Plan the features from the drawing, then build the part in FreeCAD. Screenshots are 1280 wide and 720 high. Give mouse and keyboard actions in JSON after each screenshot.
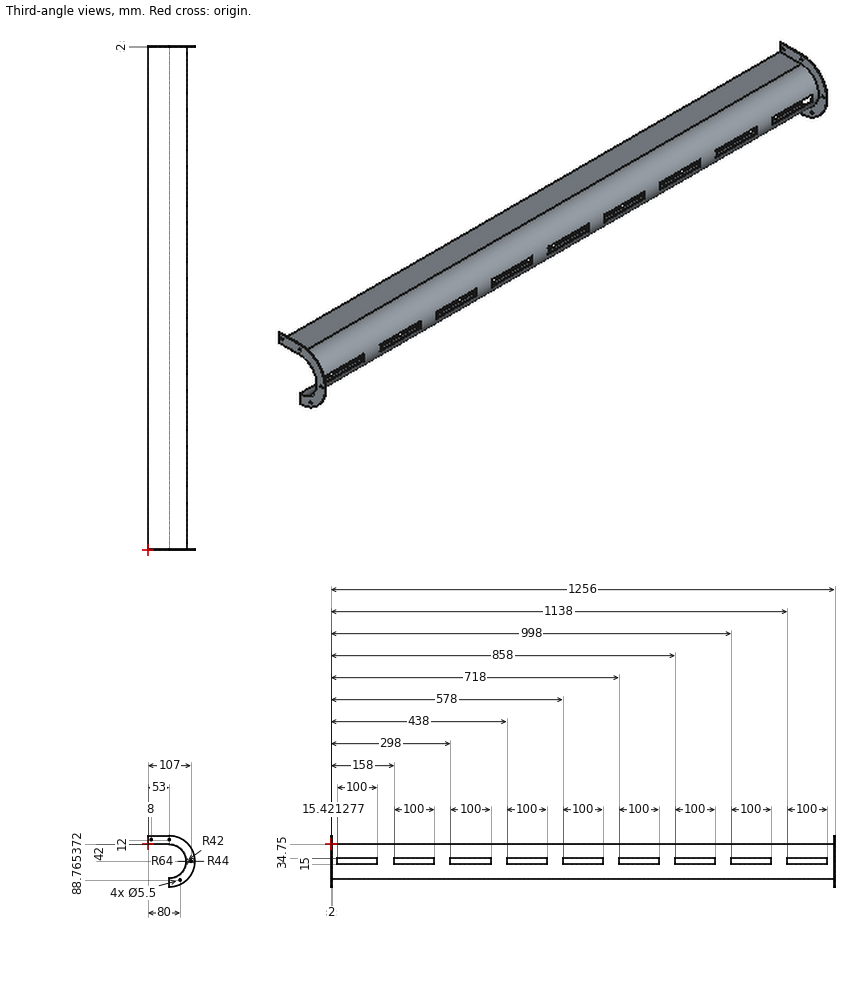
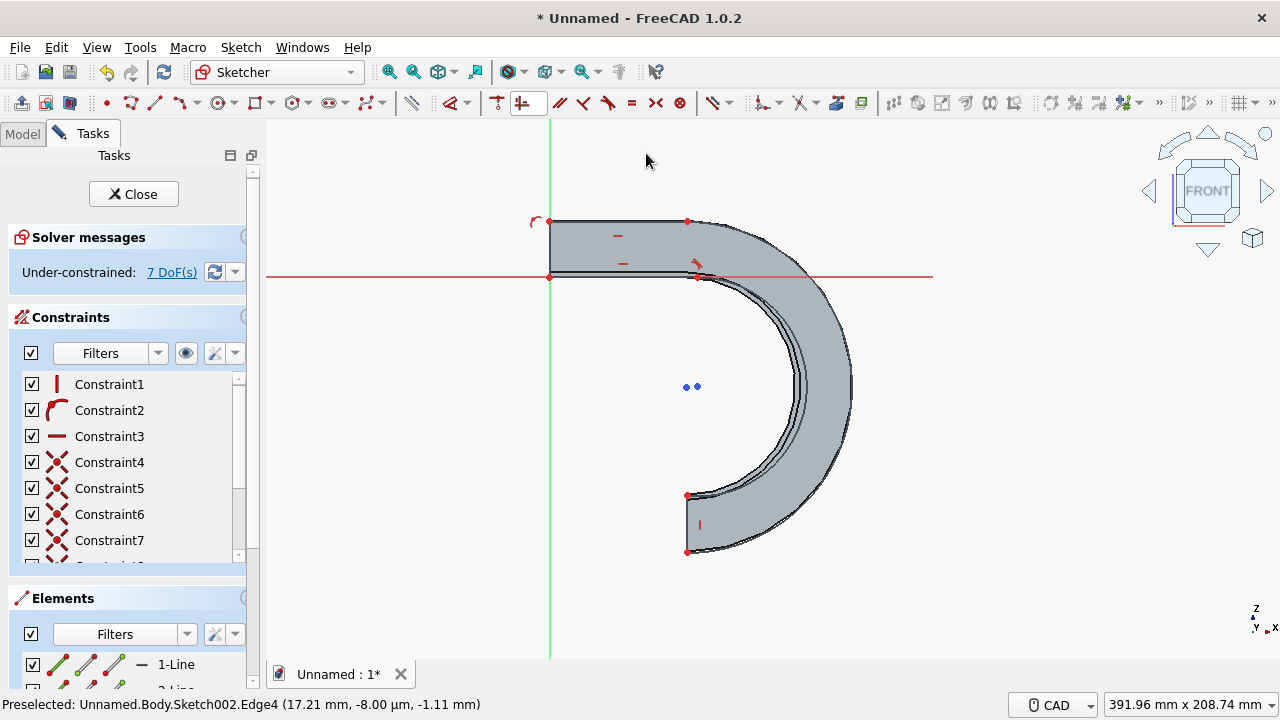
{"action": "left_click", "coordinate": [821, 485]}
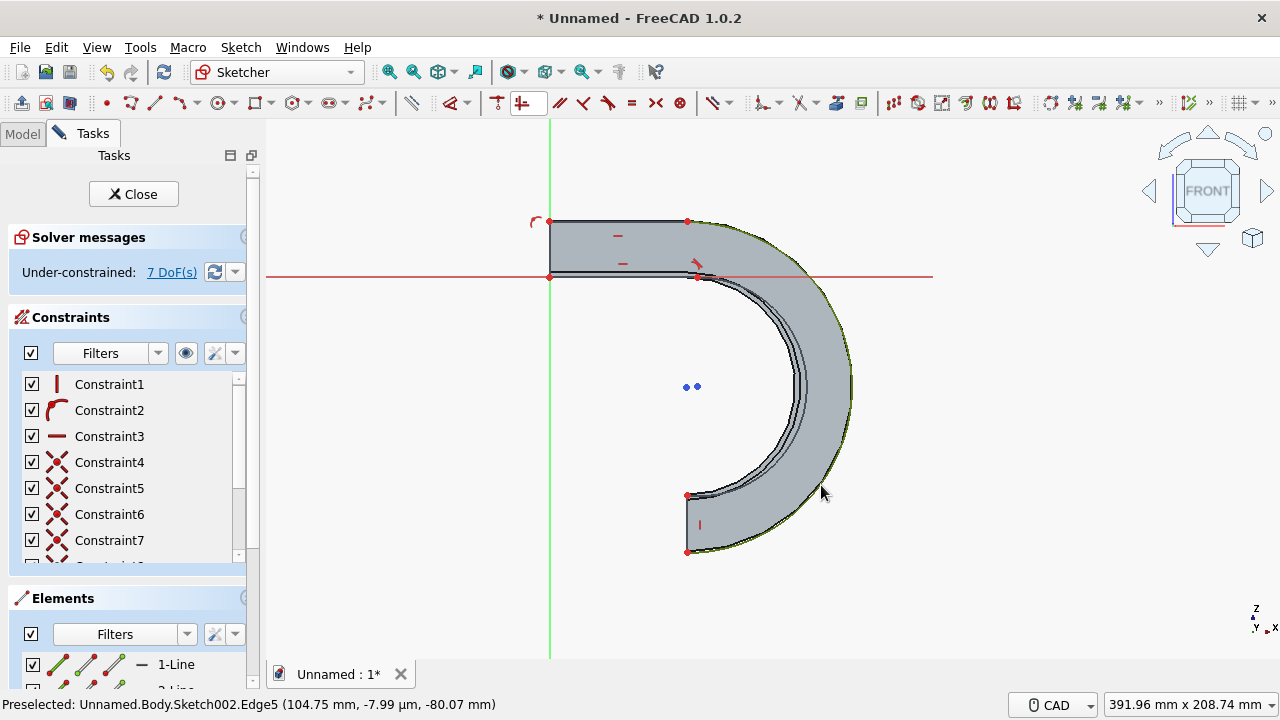
{"action": "left_click", "coordinate": [781, 457]}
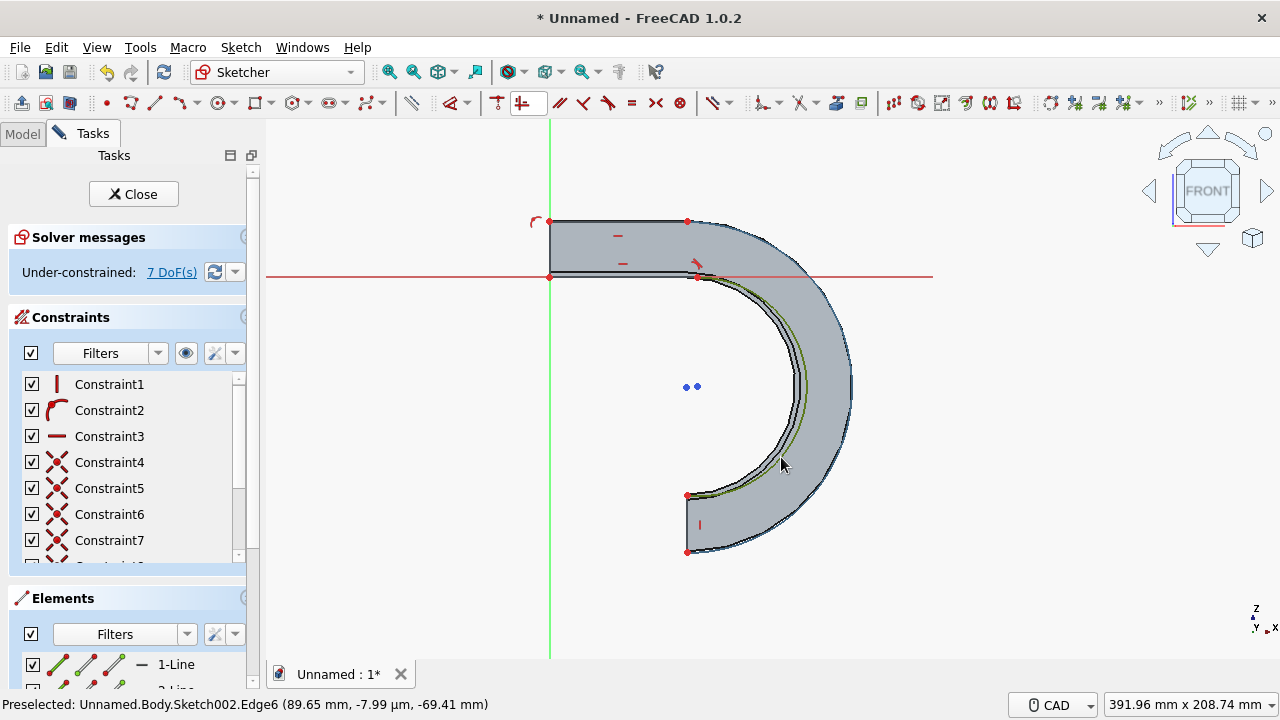
{"action": "left_click", "coordinate": [498, 104]}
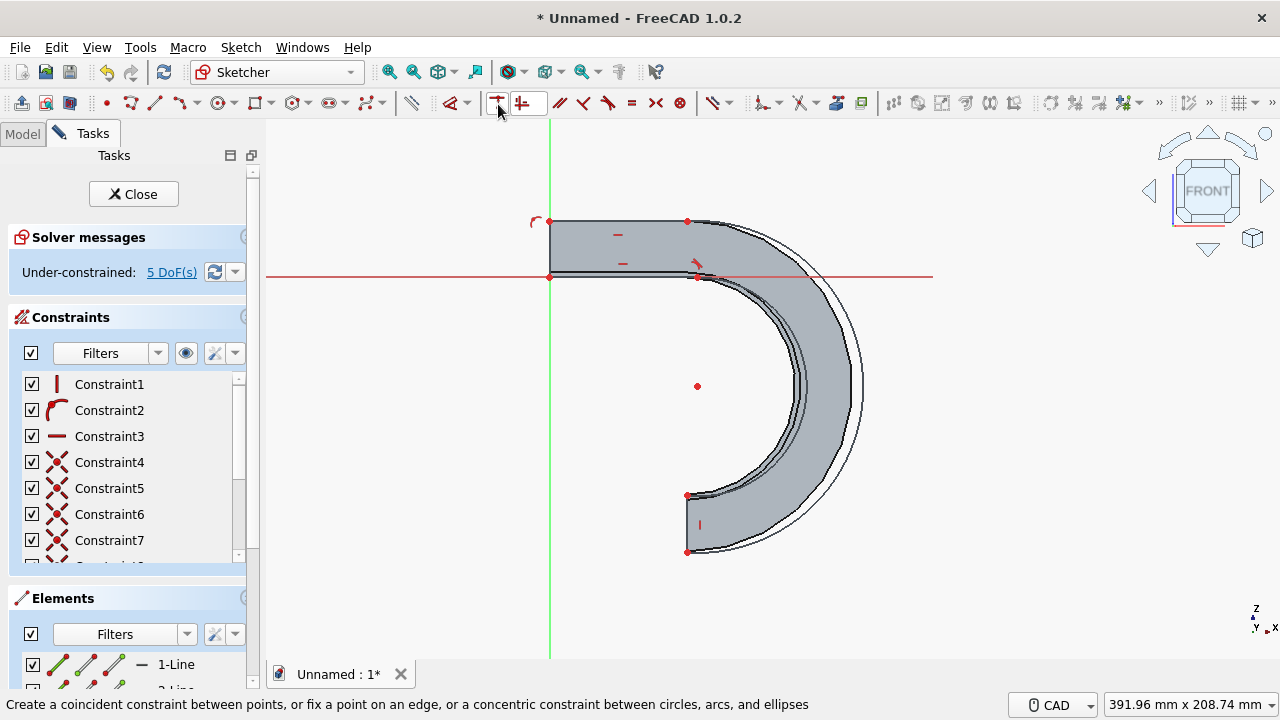
{"action": "key", "text": "d"}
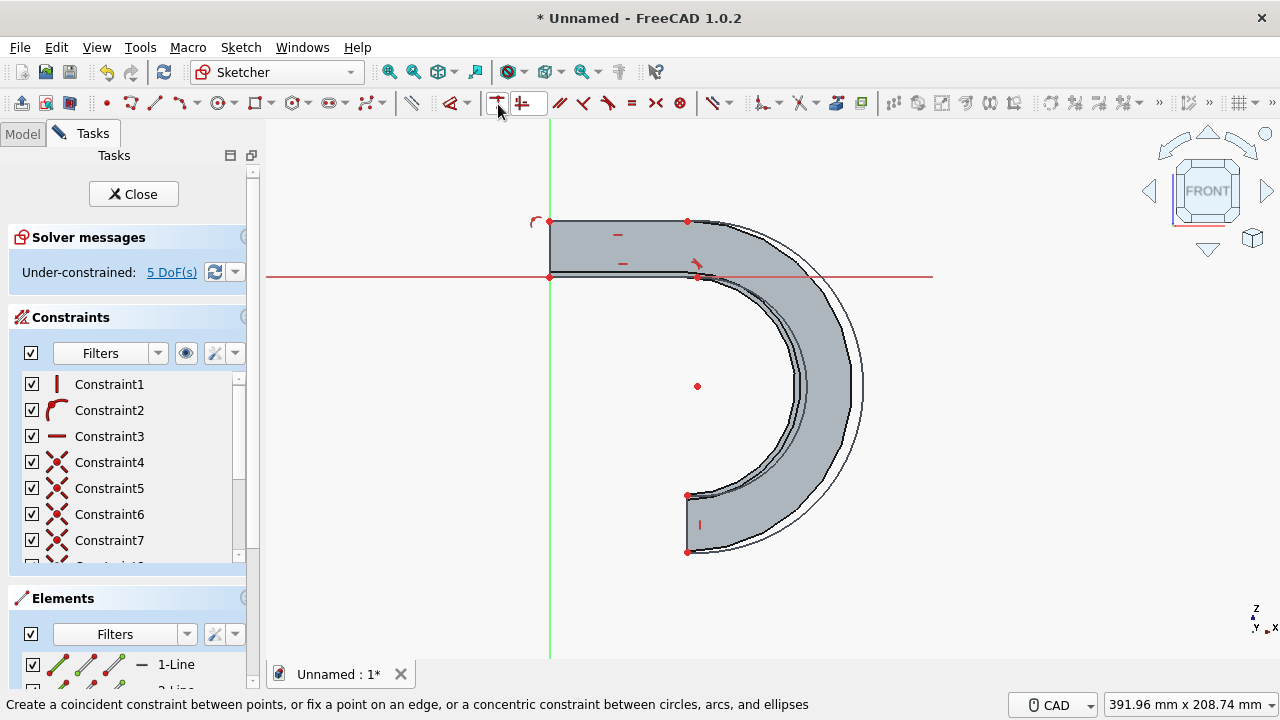
{"action": "left_click", "coordinate": [829, 488]}
{"action": "left_click", "coordinate": [854, 507]}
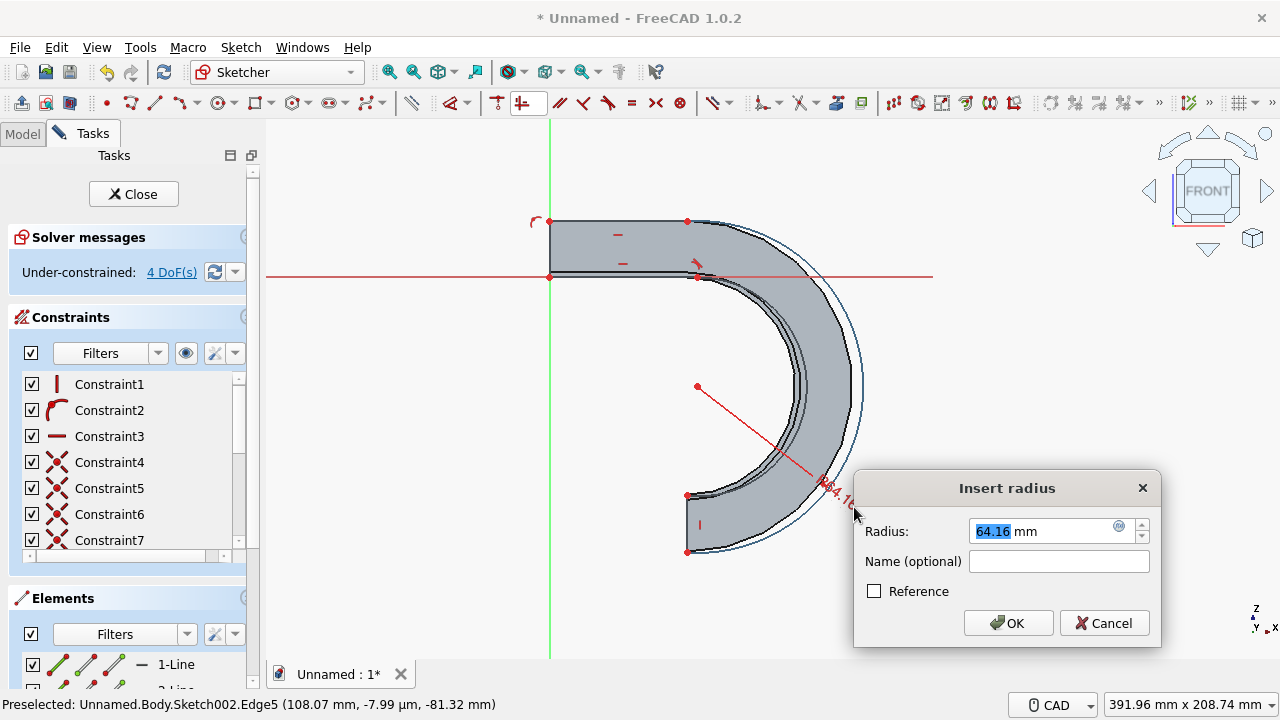
{"action": "type", "text": "64"}
{"action": "key", "text": "Return"}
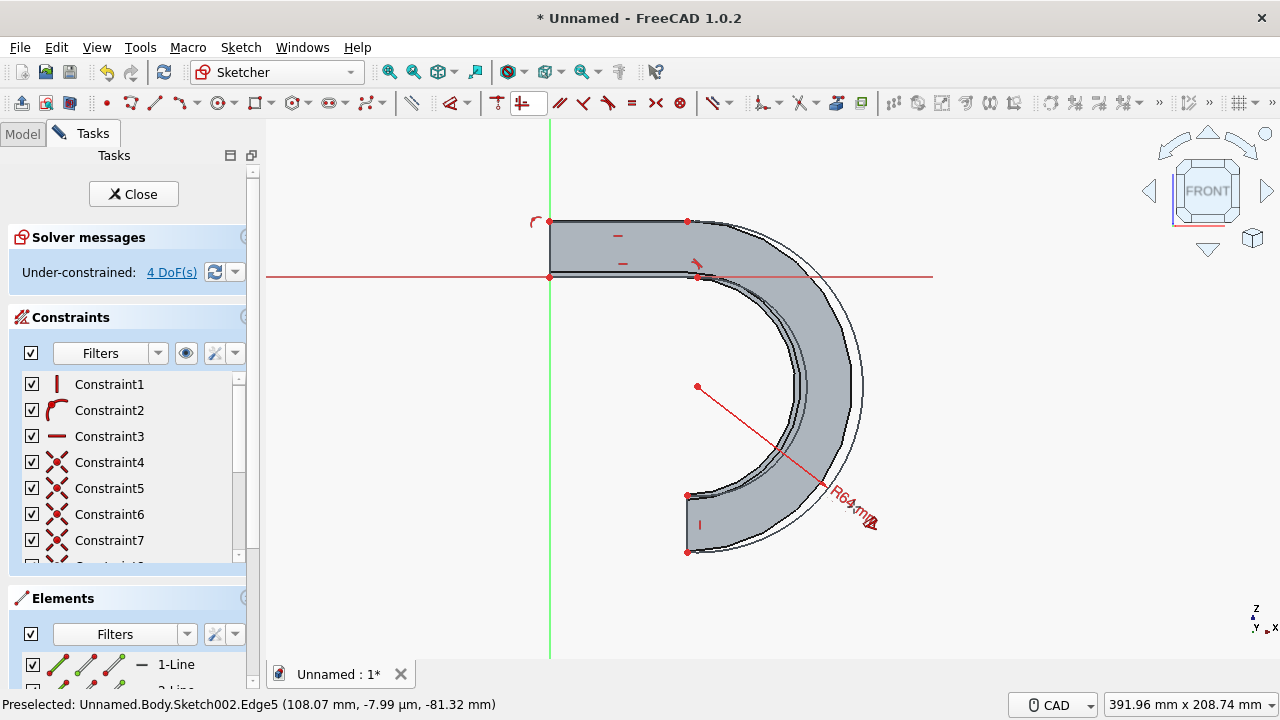
{"action": "left_click", "coordinate": [781, 457]}
{"action": "left_click", "coordinate": [806, 478]}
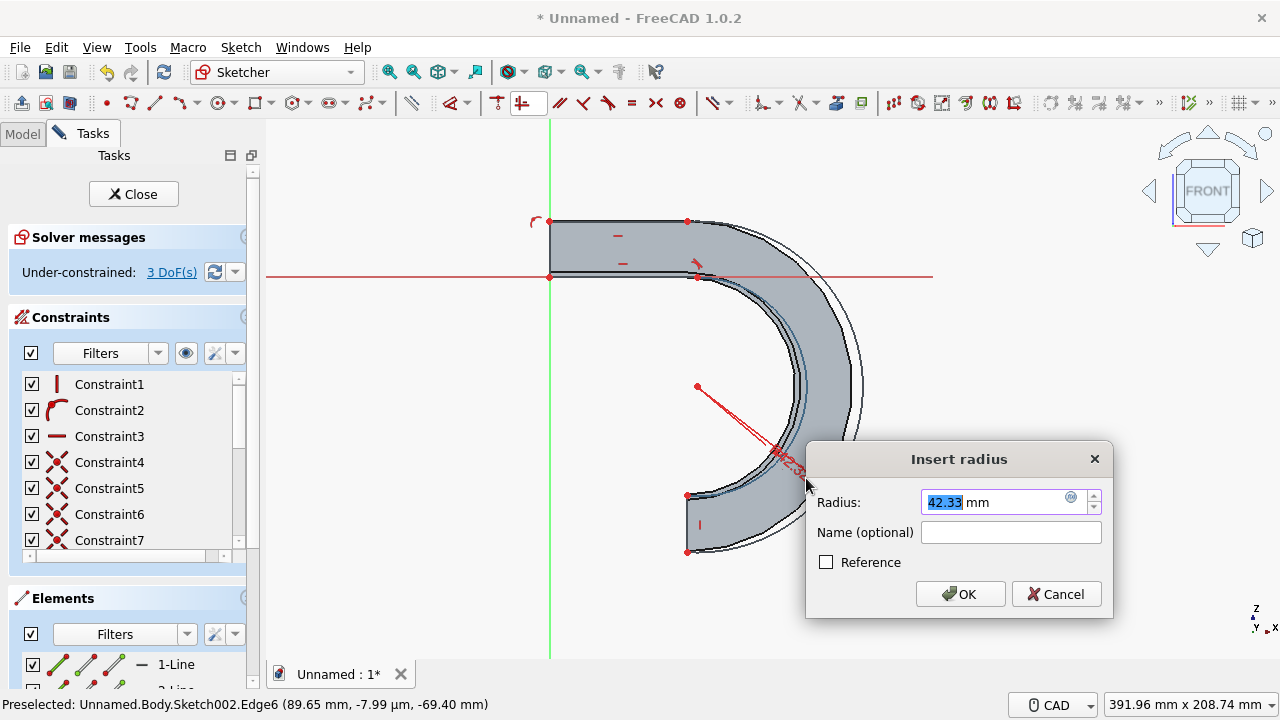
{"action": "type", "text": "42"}
{"action": "key", "text": "Return"}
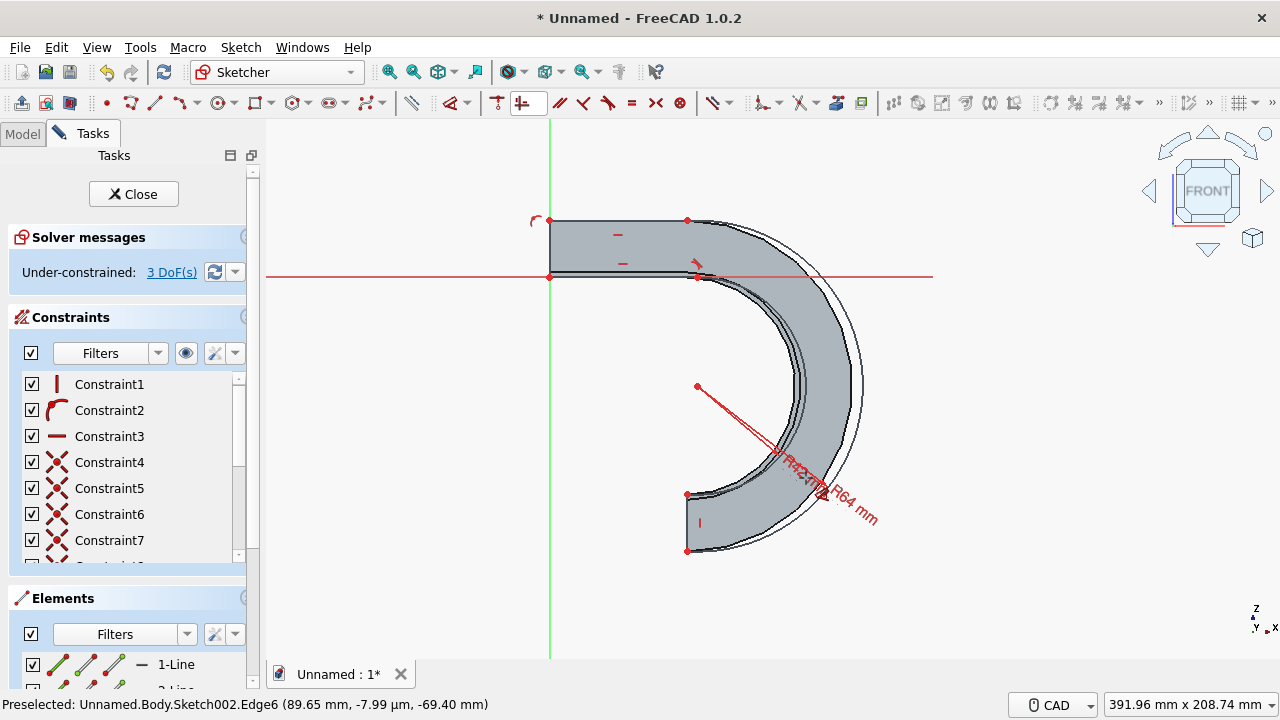
{"action": "left_click", "coordinate": [646, 221]}
{"action": "left_click", "coordinate": [618, 187]}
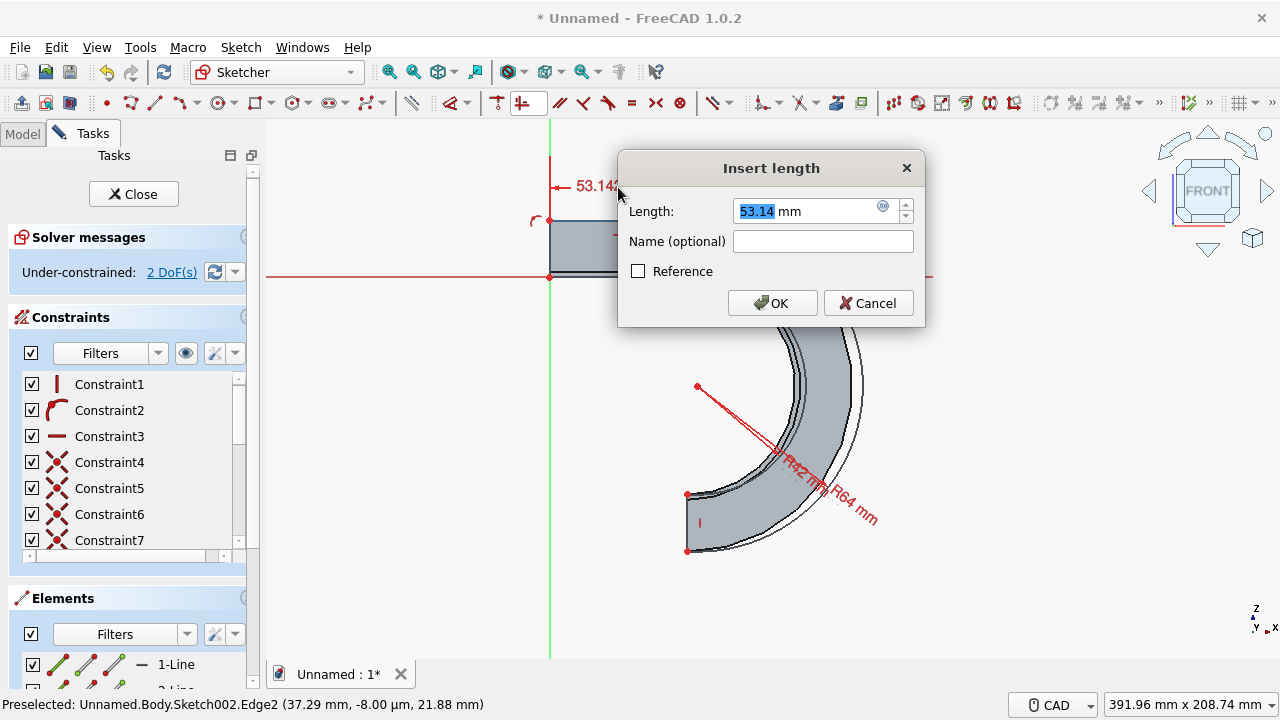
{"action": "type", "text": "53"}
{"action": "key", "text": "Return"}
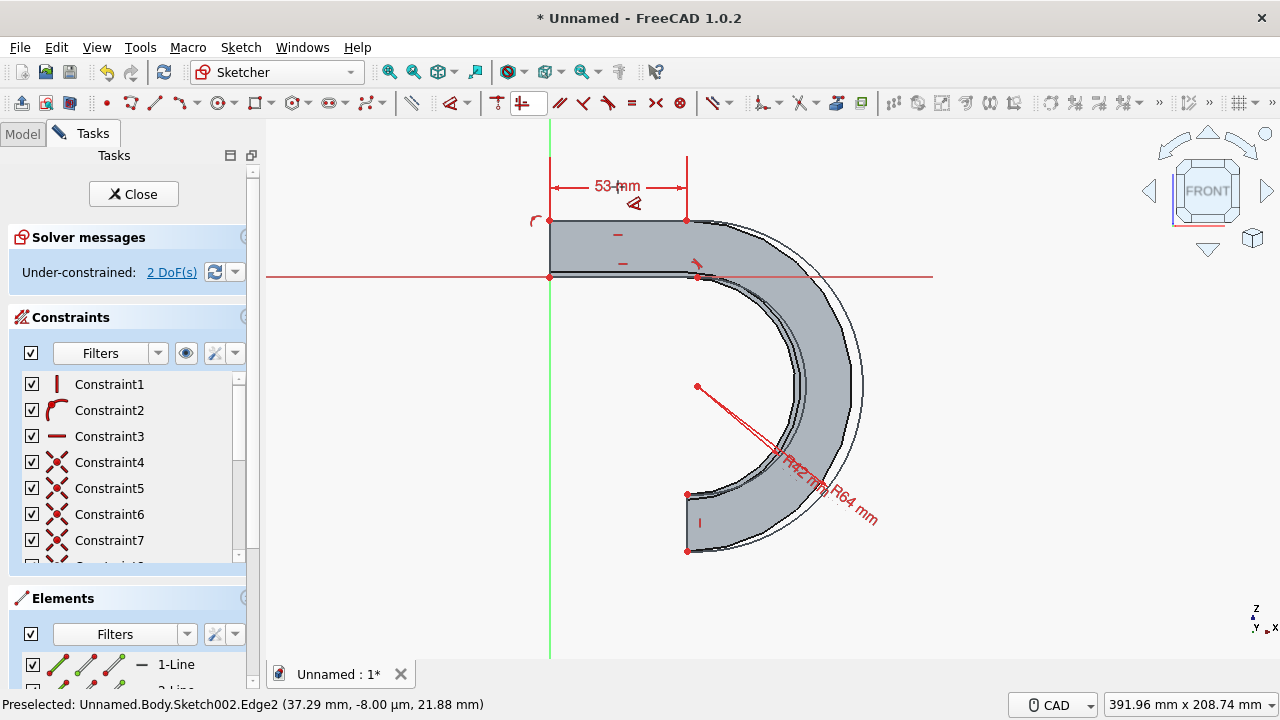
{"action": "left_click", "coordinate": [594, 277]}
{"action": "left_click", "coordinate": [623, 243]}